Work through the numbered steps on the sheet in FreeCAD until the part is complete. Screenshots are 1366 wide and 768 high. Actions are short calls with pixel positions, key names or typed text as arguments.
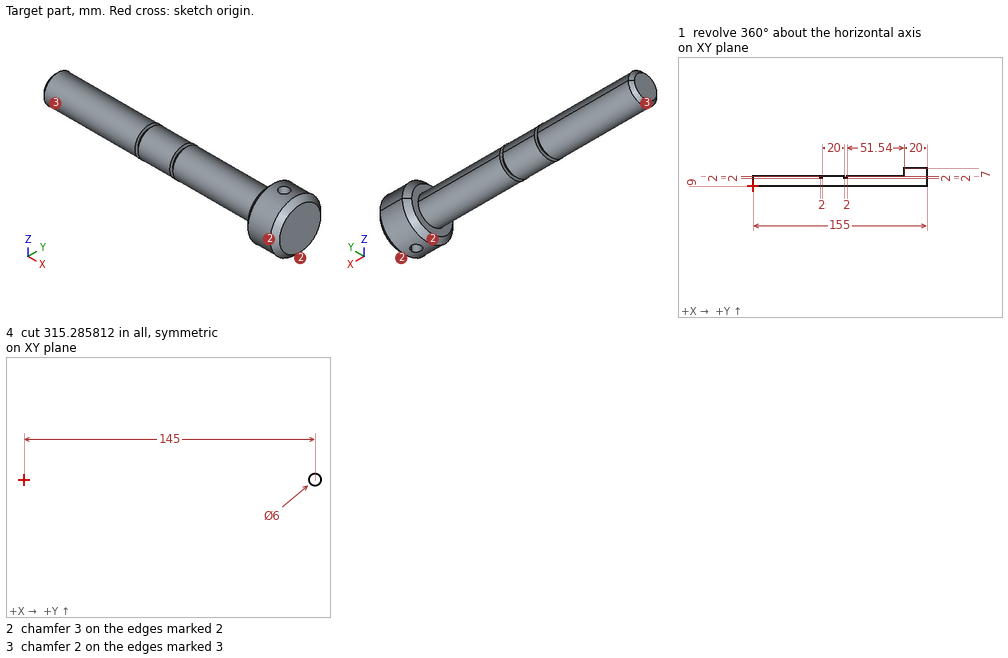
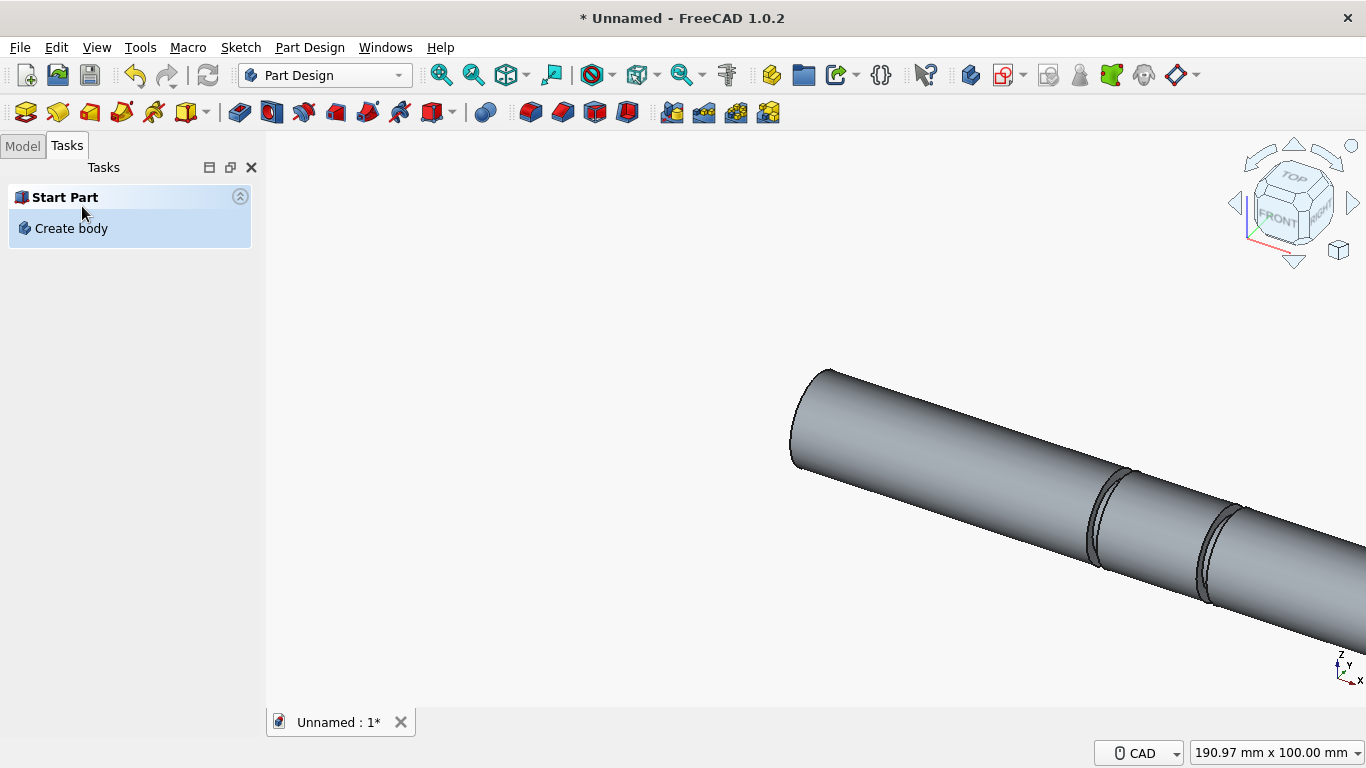
click(442, 76)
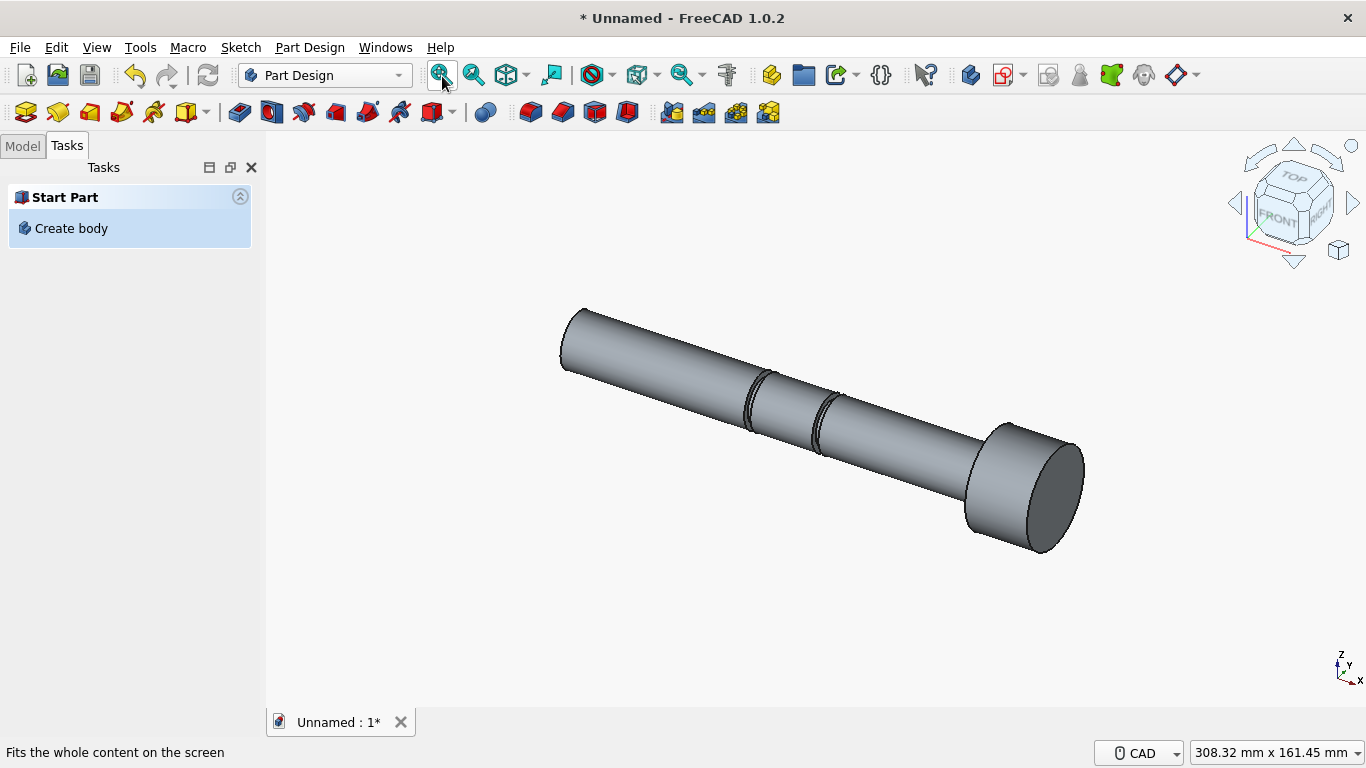
click(1027, 526)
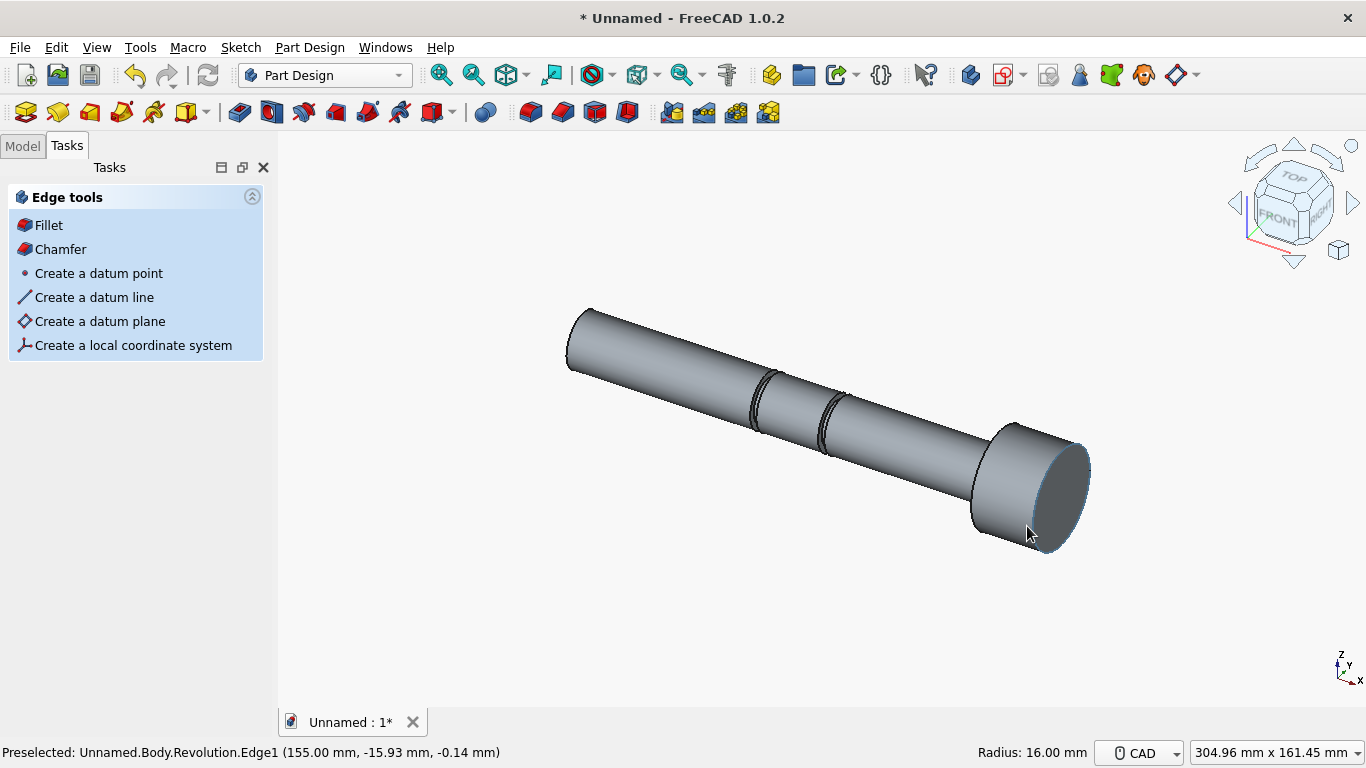
key(0)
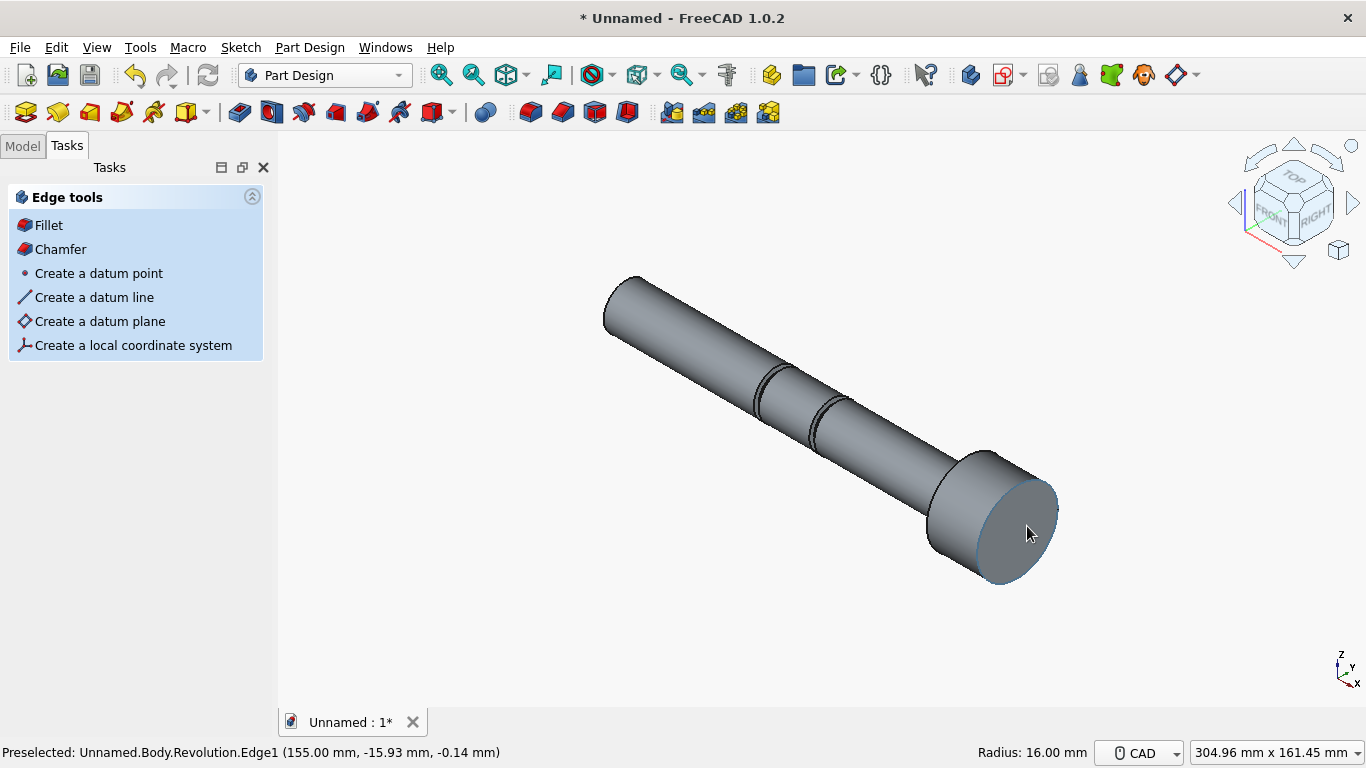
click(979, 450, ctrl)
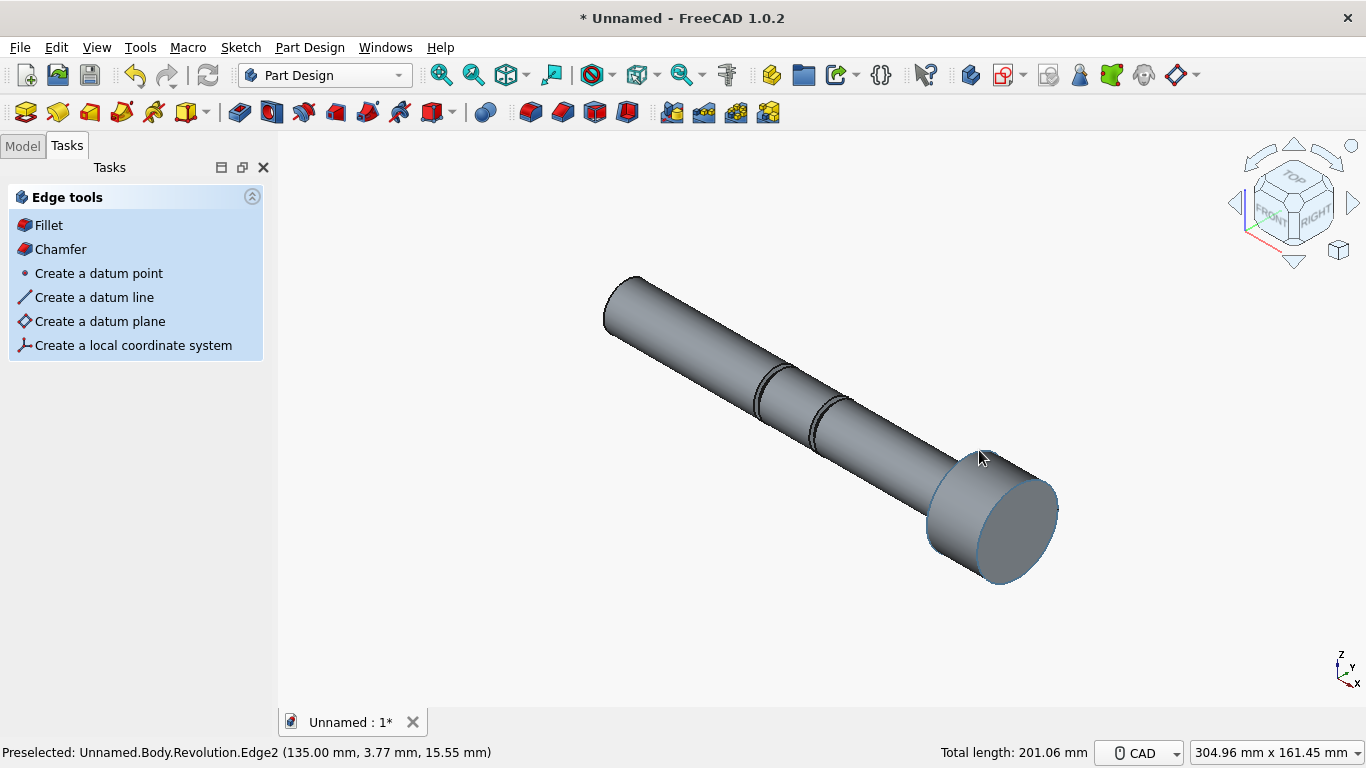
click(564, 112)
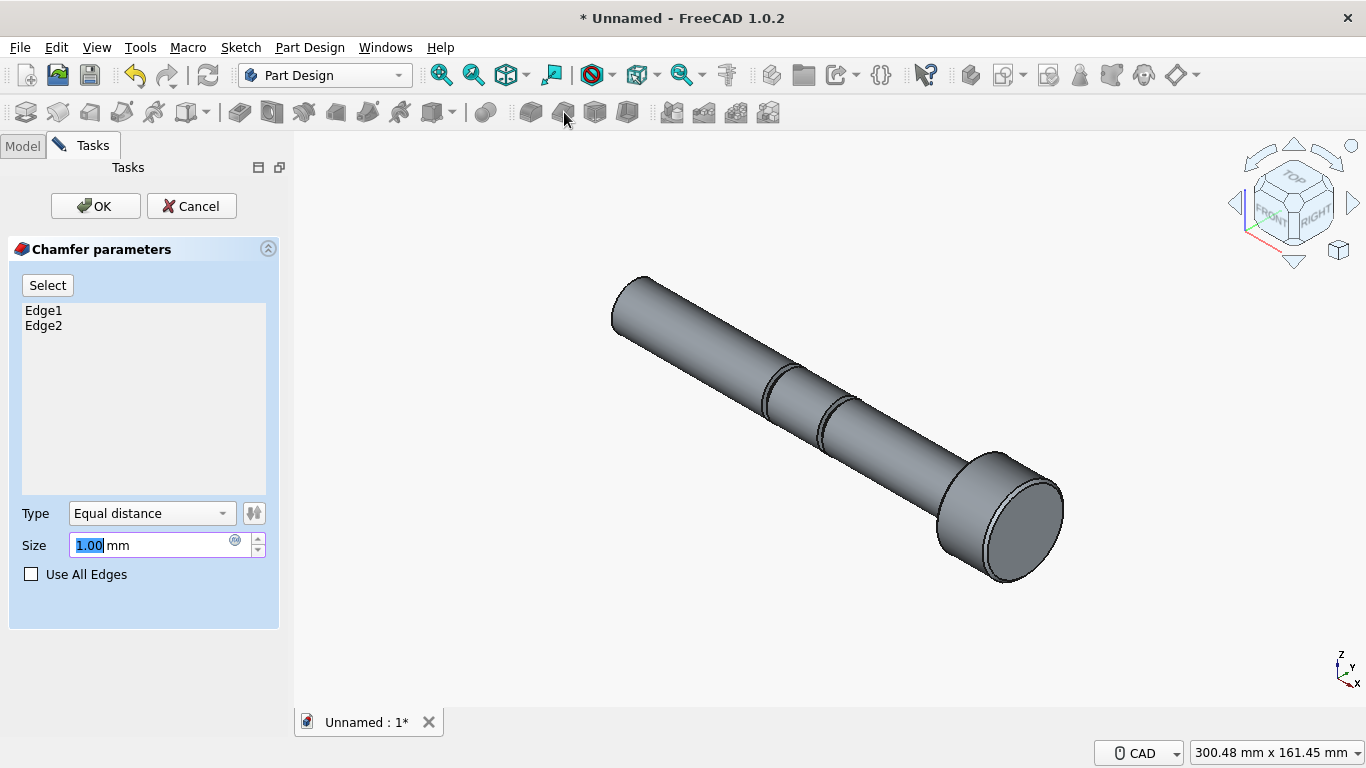
text(3)
key(Tab)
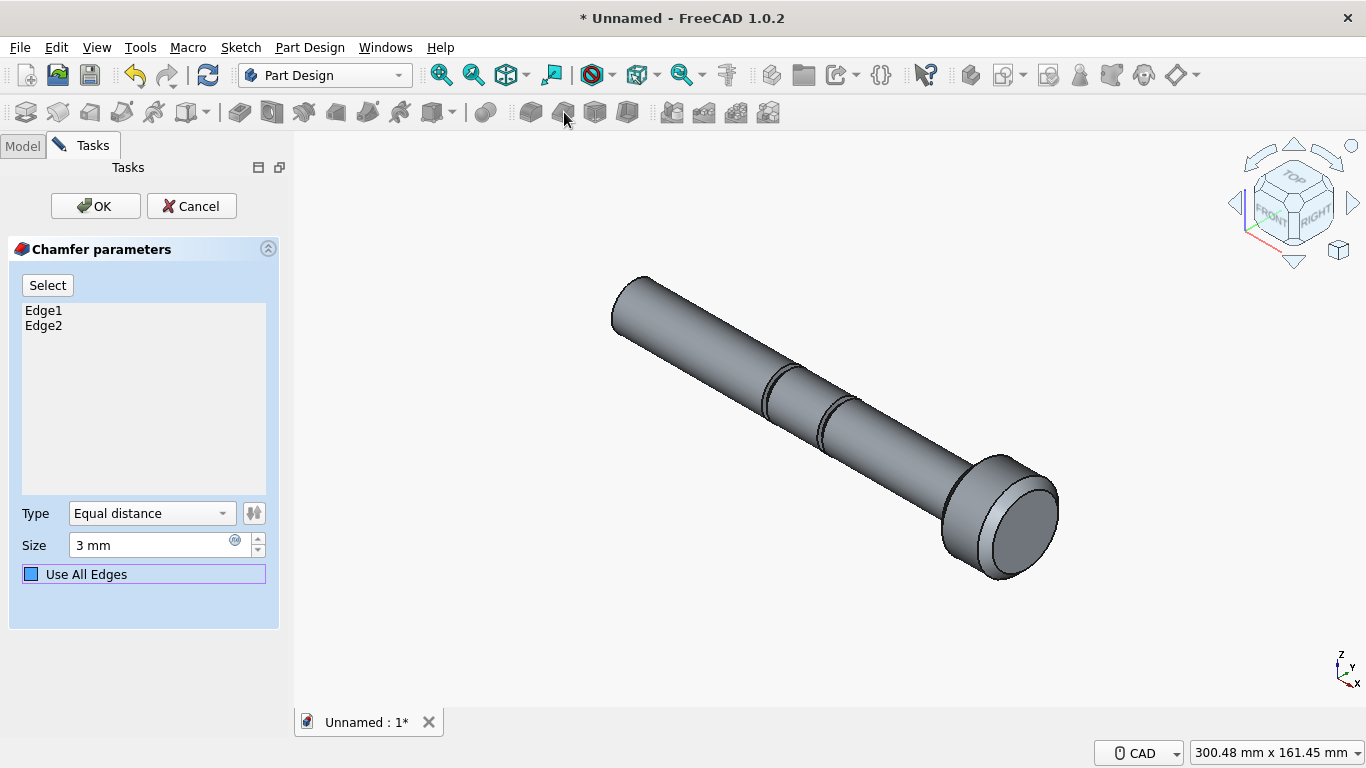
click(96, 206)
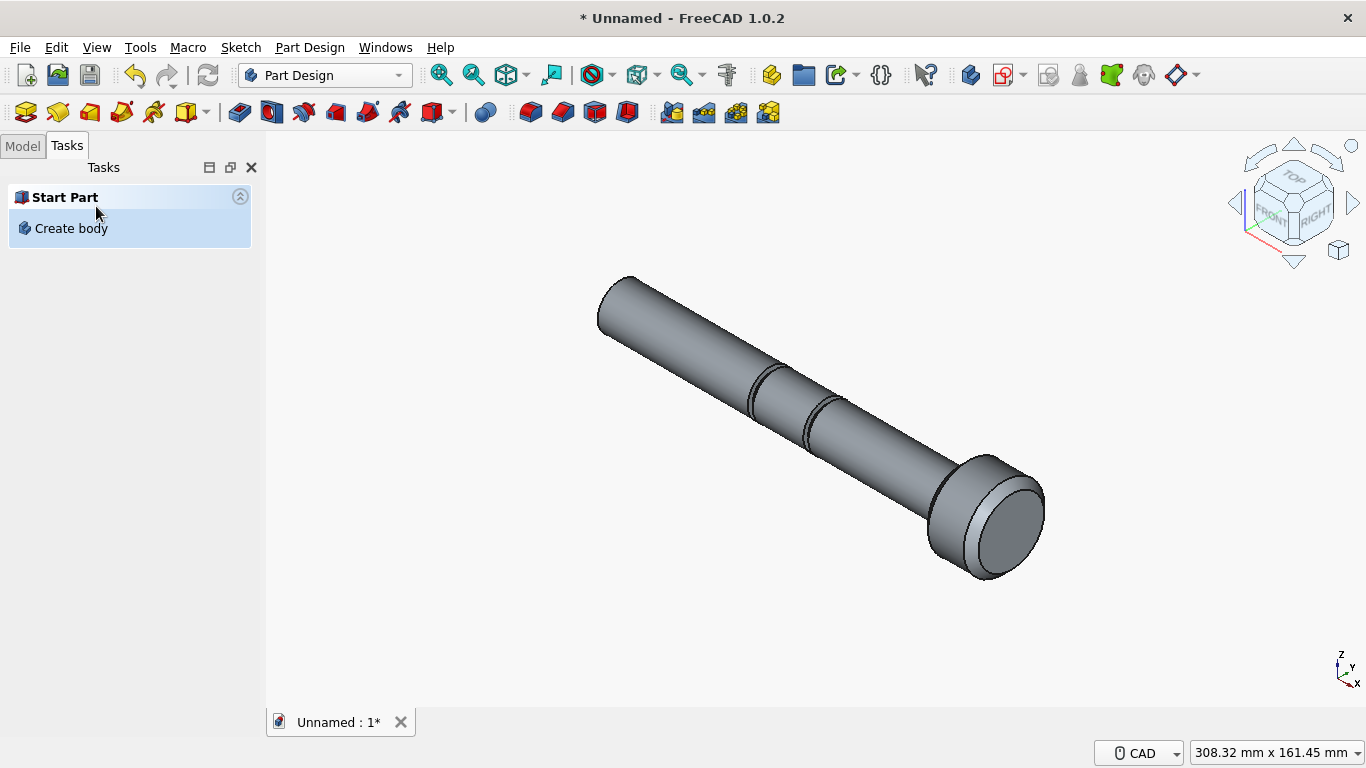
key(2)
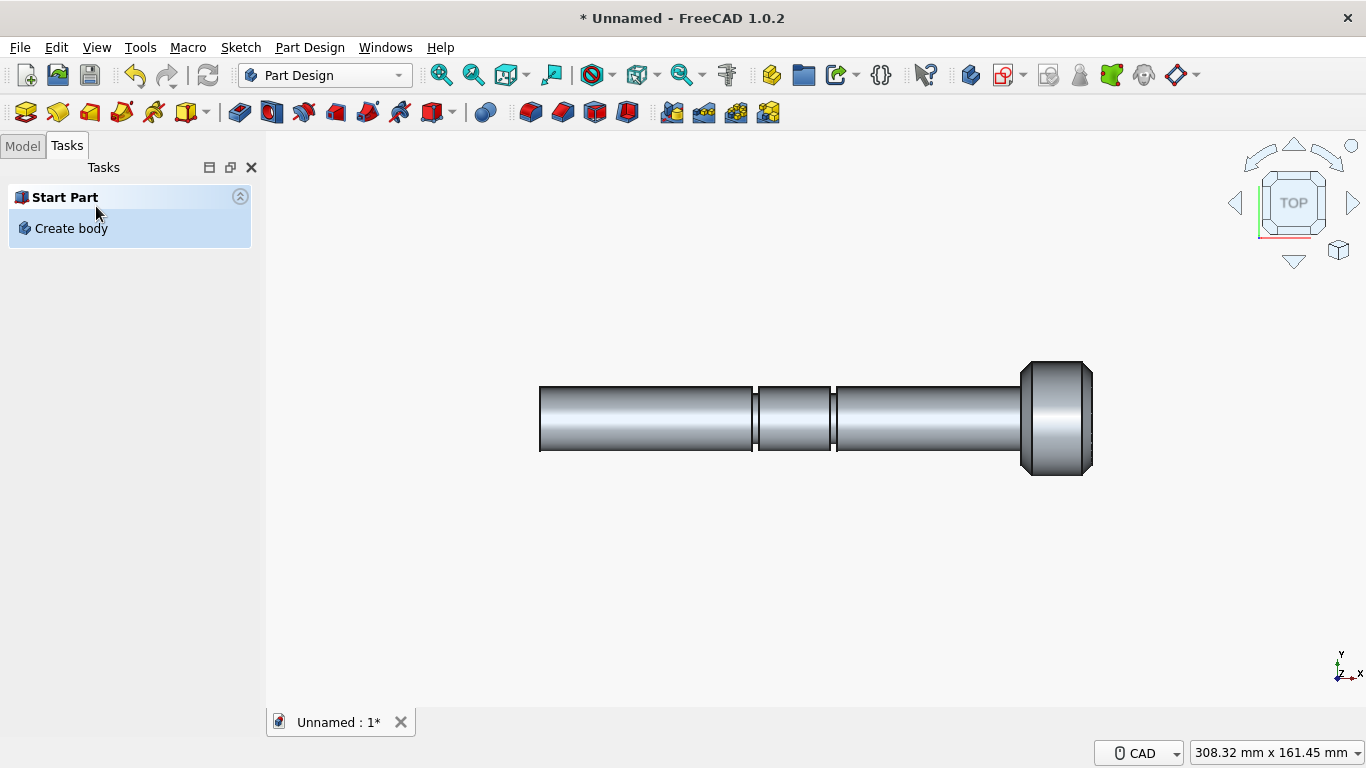
click(540, 444)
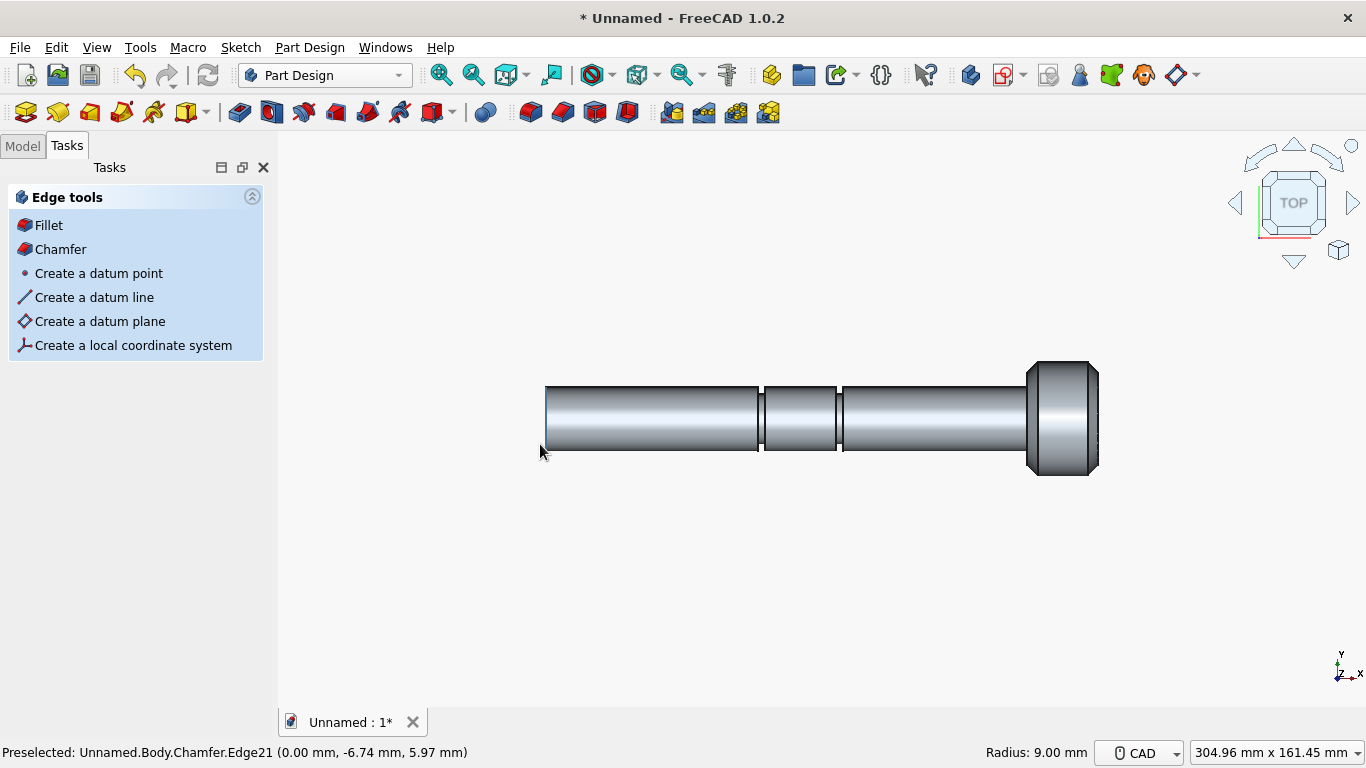
click(564, 112)